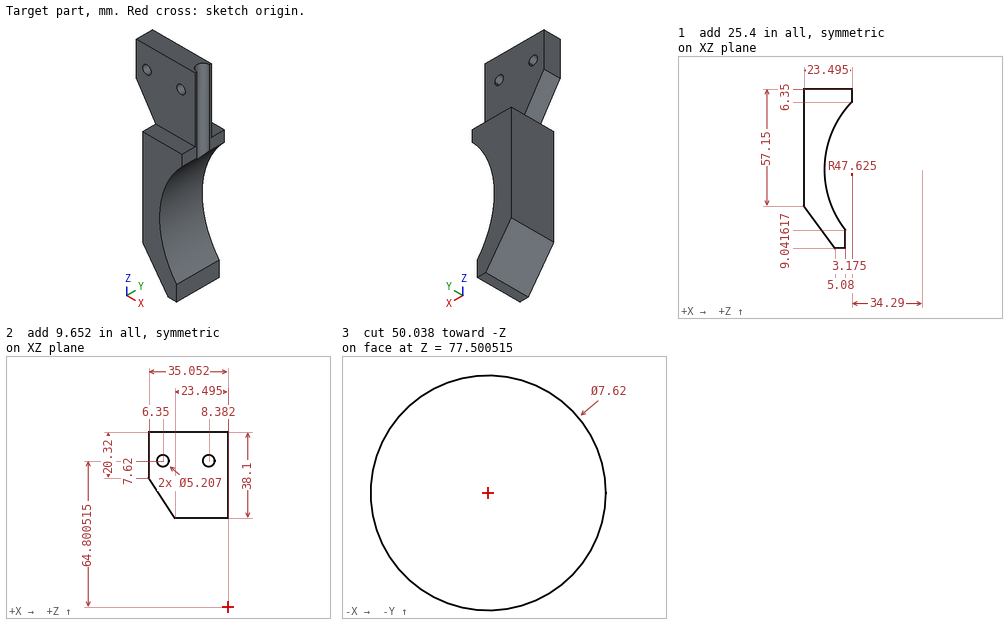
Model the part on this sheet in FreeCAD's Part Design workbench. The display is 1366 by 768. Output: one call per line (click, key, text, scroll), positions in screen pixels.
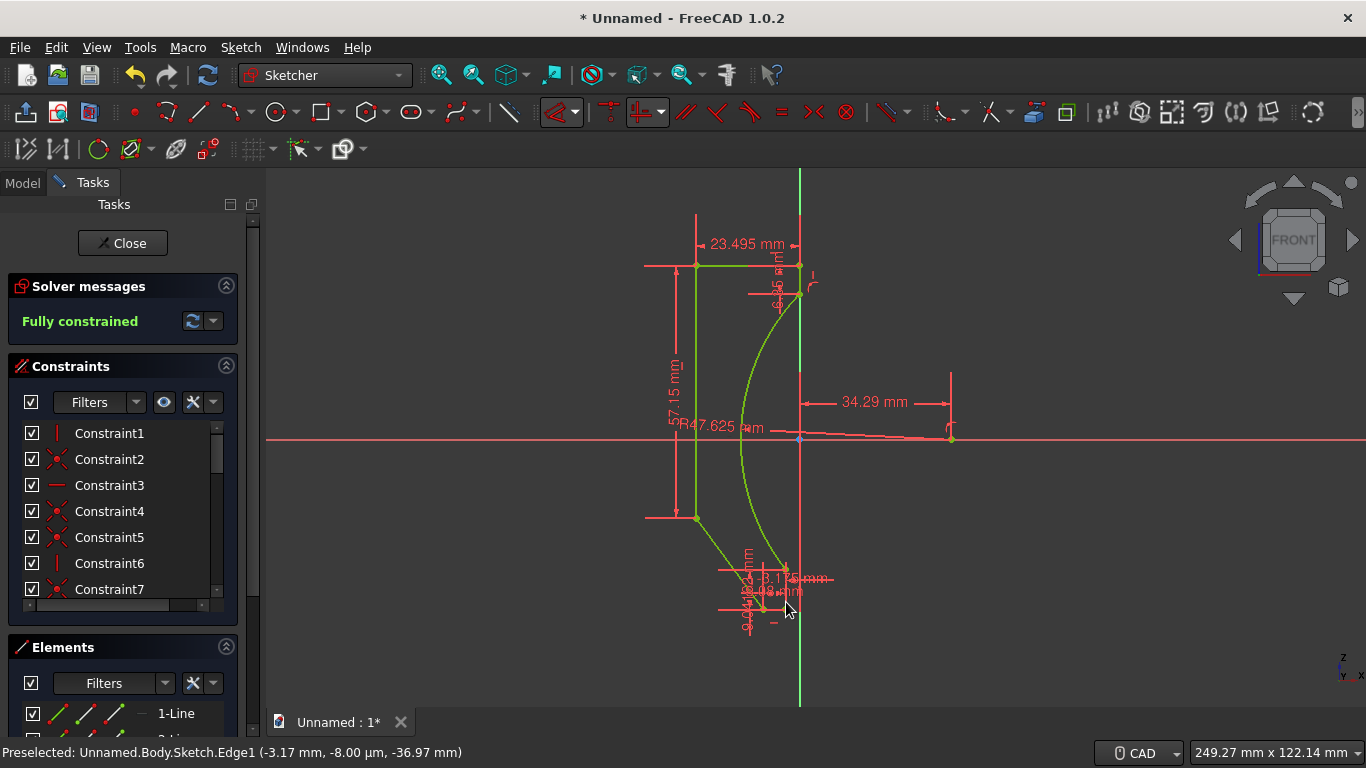
click(123, 243)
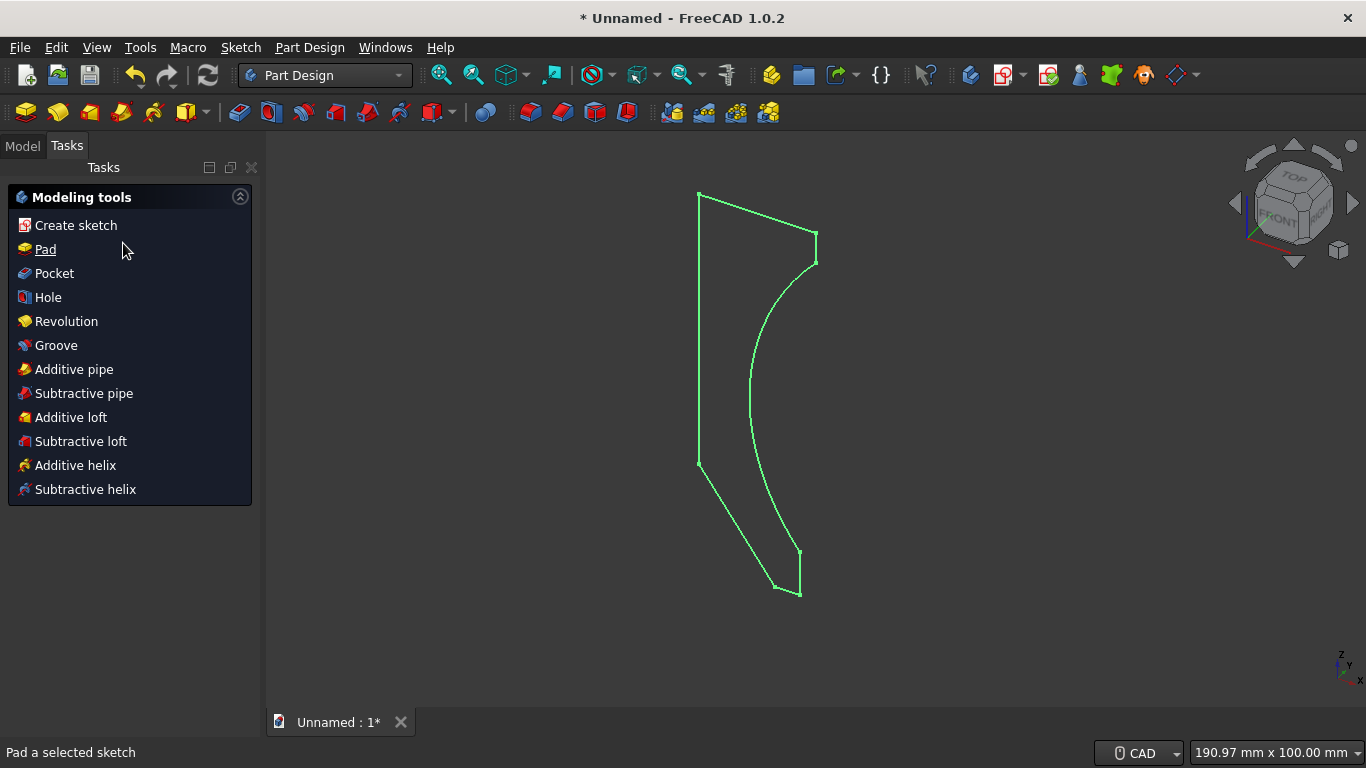
click(26, 112)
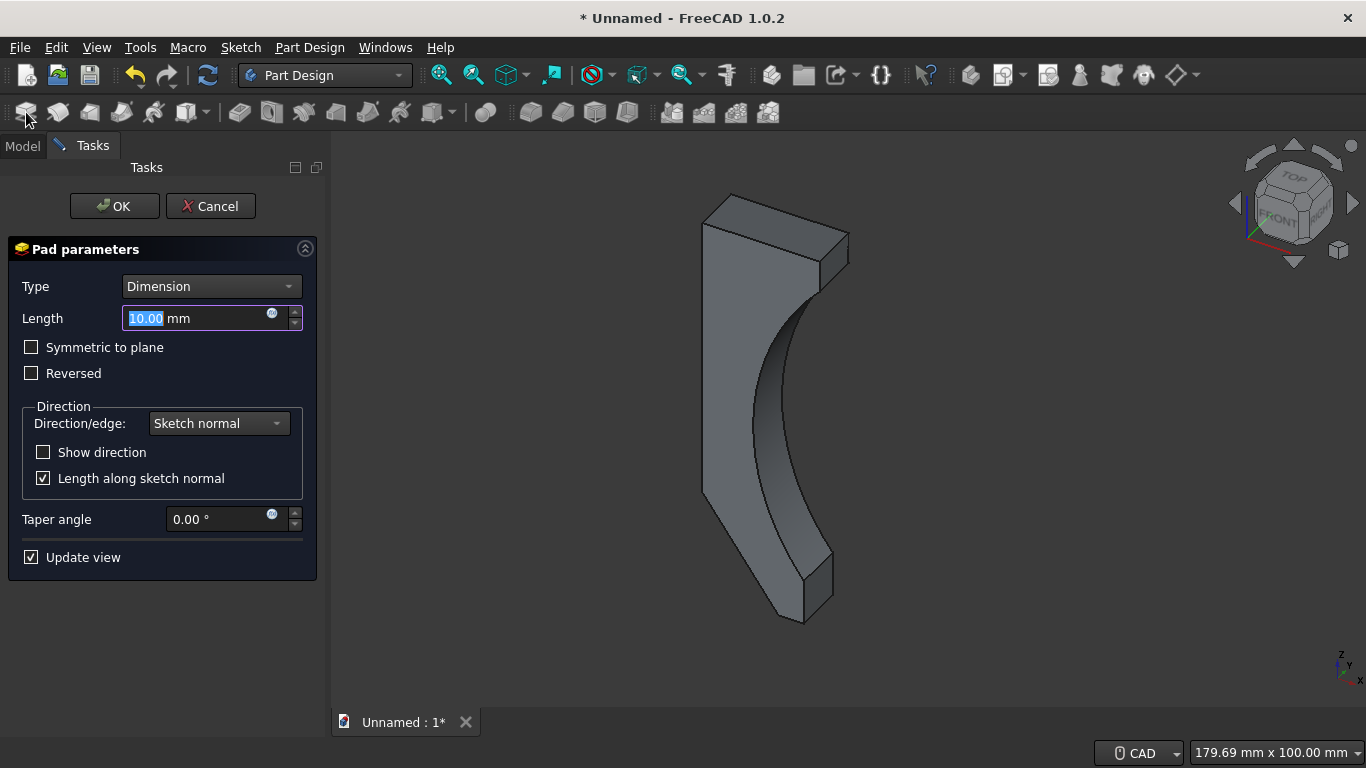
text(25.4)
key(Tab)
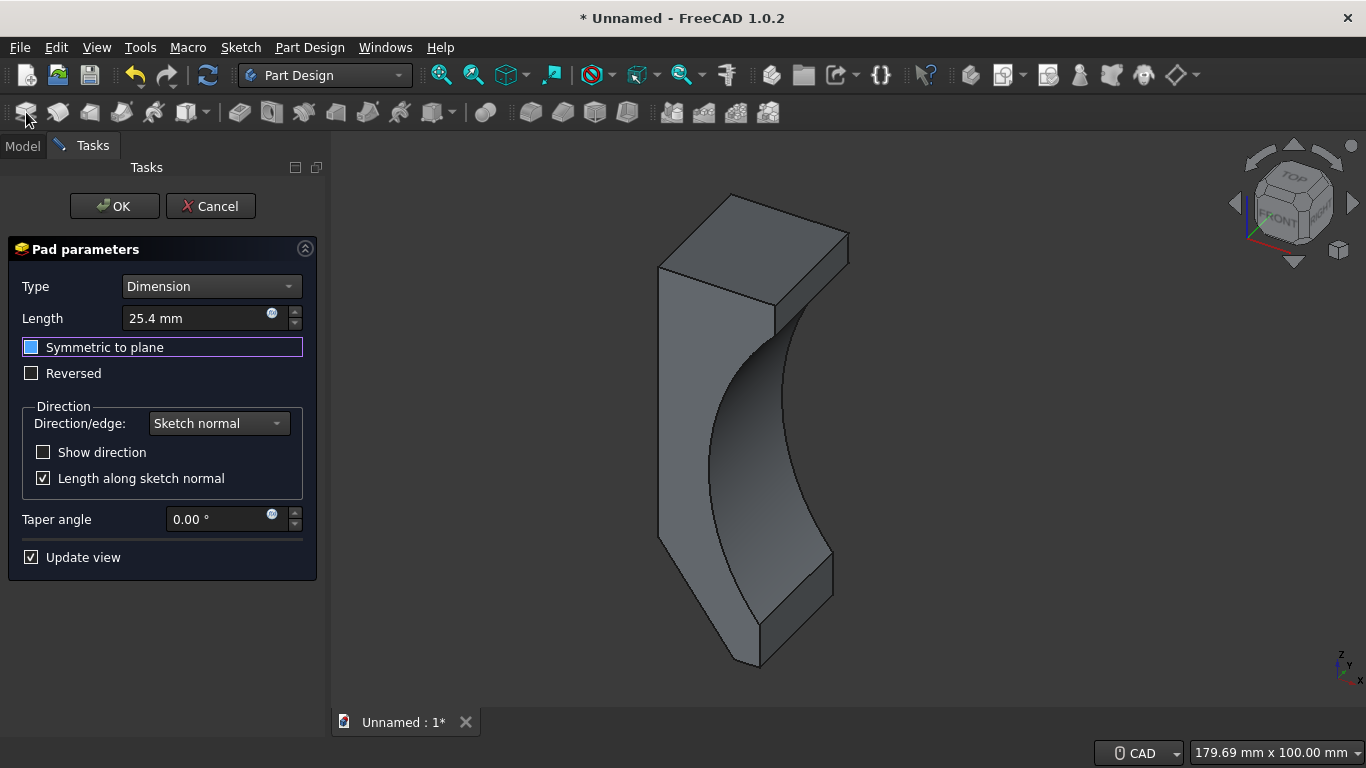
click(30, 347)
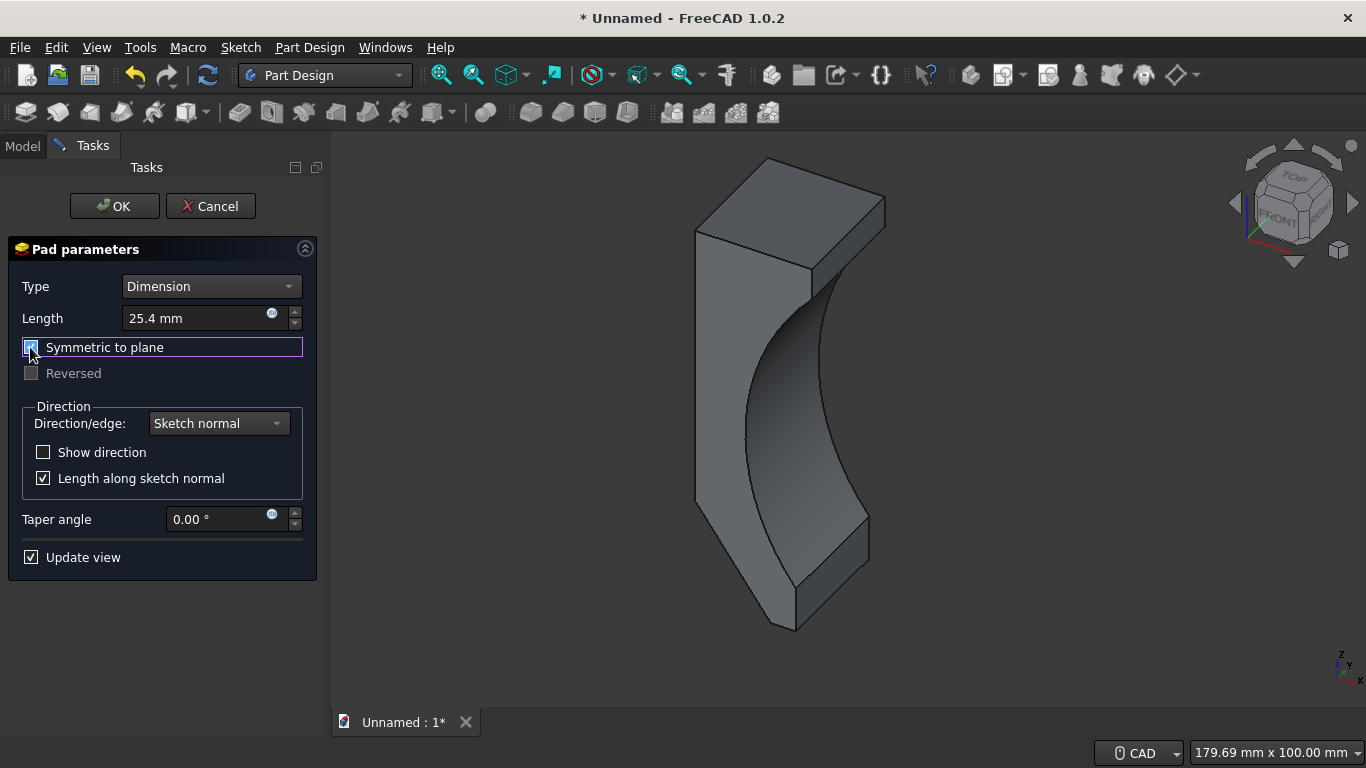
click(115, 206)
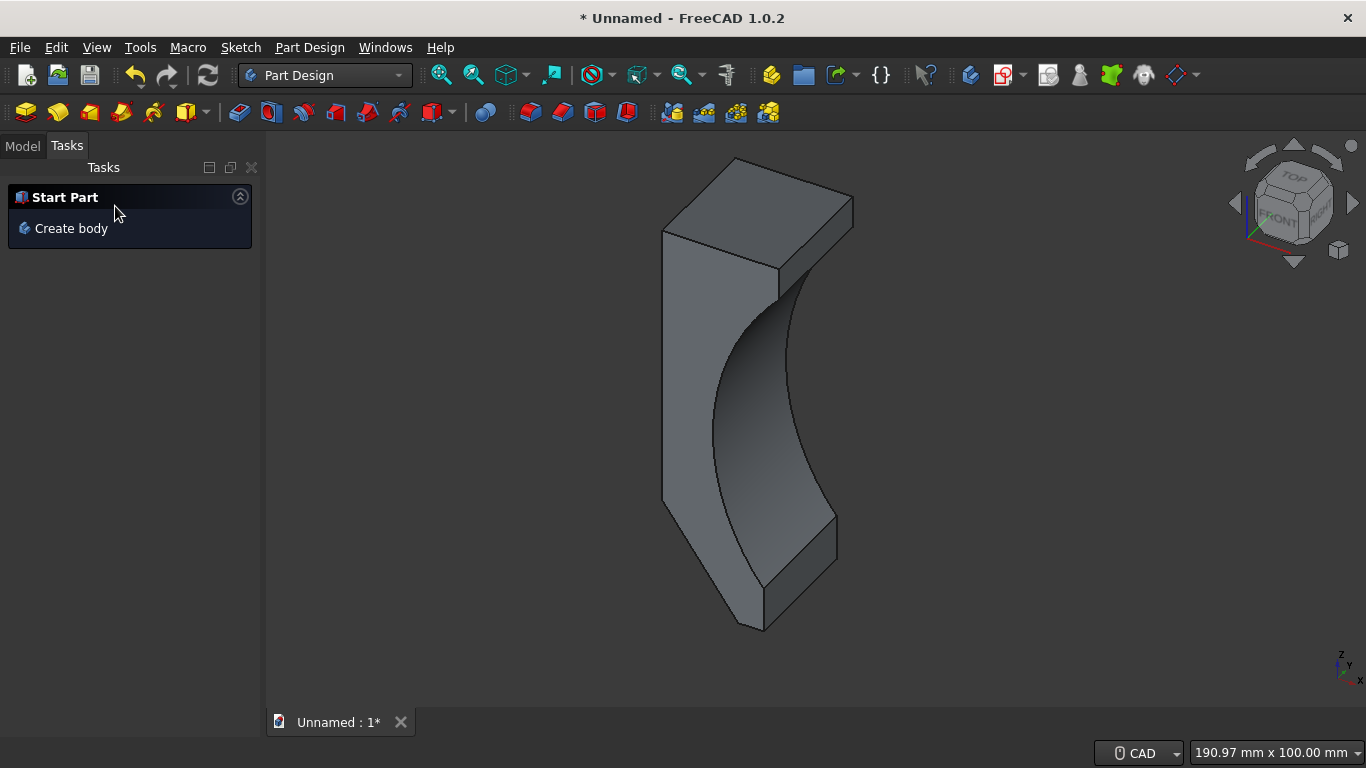
click(1004, 76)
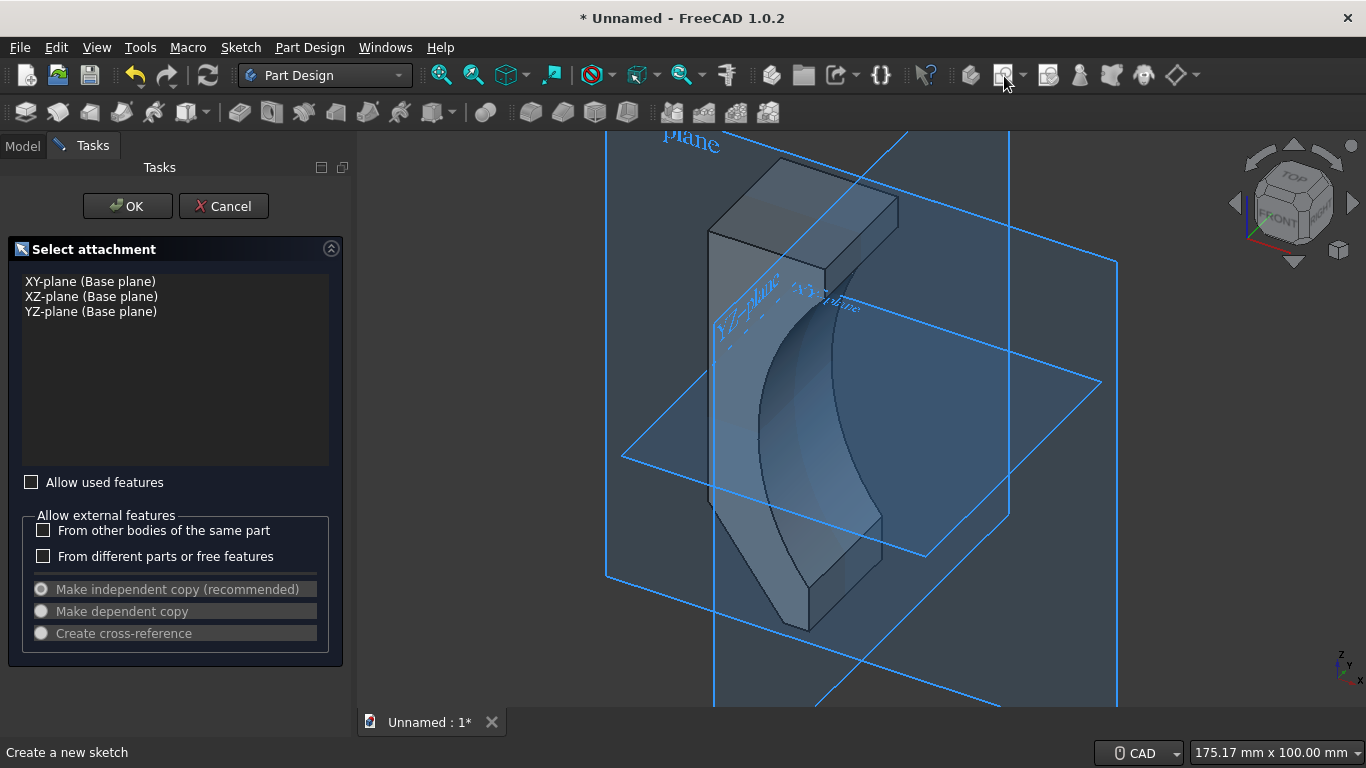
click(82, 296)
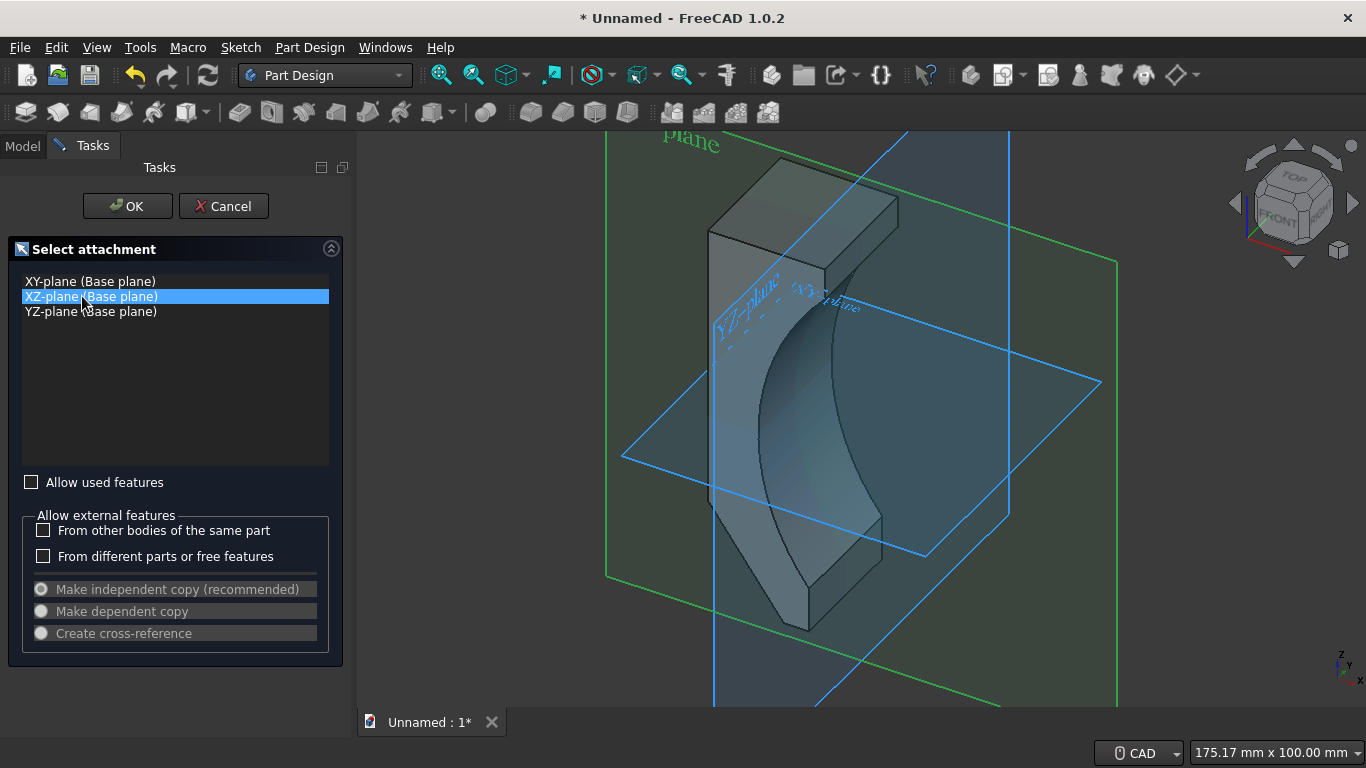
click(128, 206)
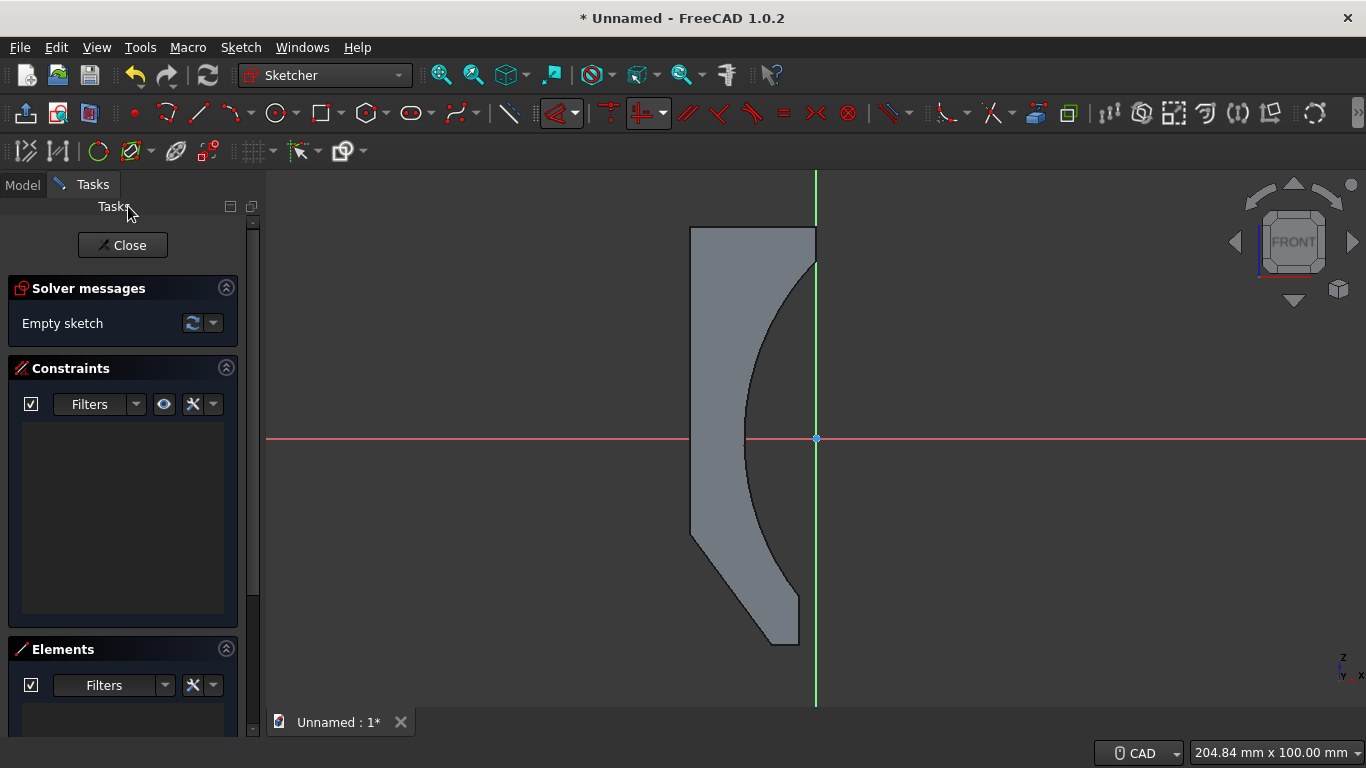
click(90, 114)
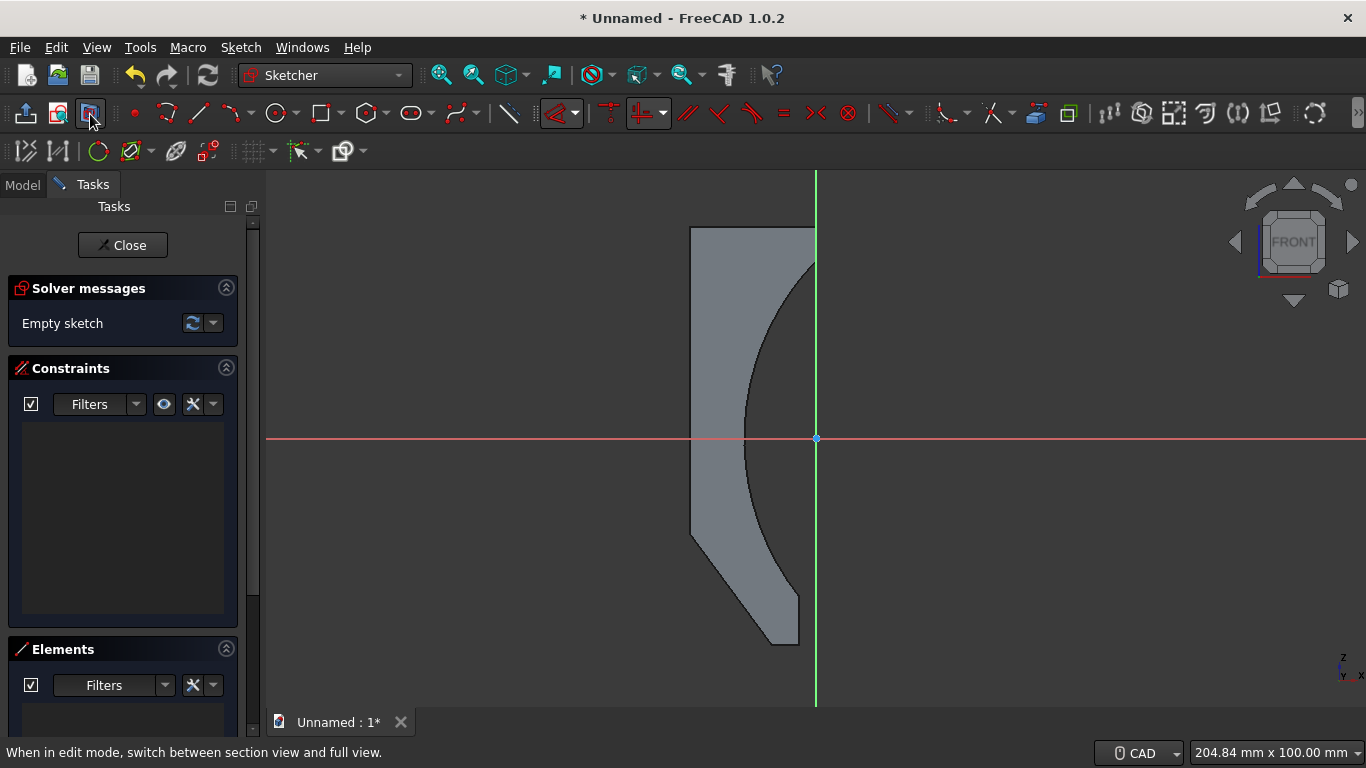
scroll(800, 679, down, 2)